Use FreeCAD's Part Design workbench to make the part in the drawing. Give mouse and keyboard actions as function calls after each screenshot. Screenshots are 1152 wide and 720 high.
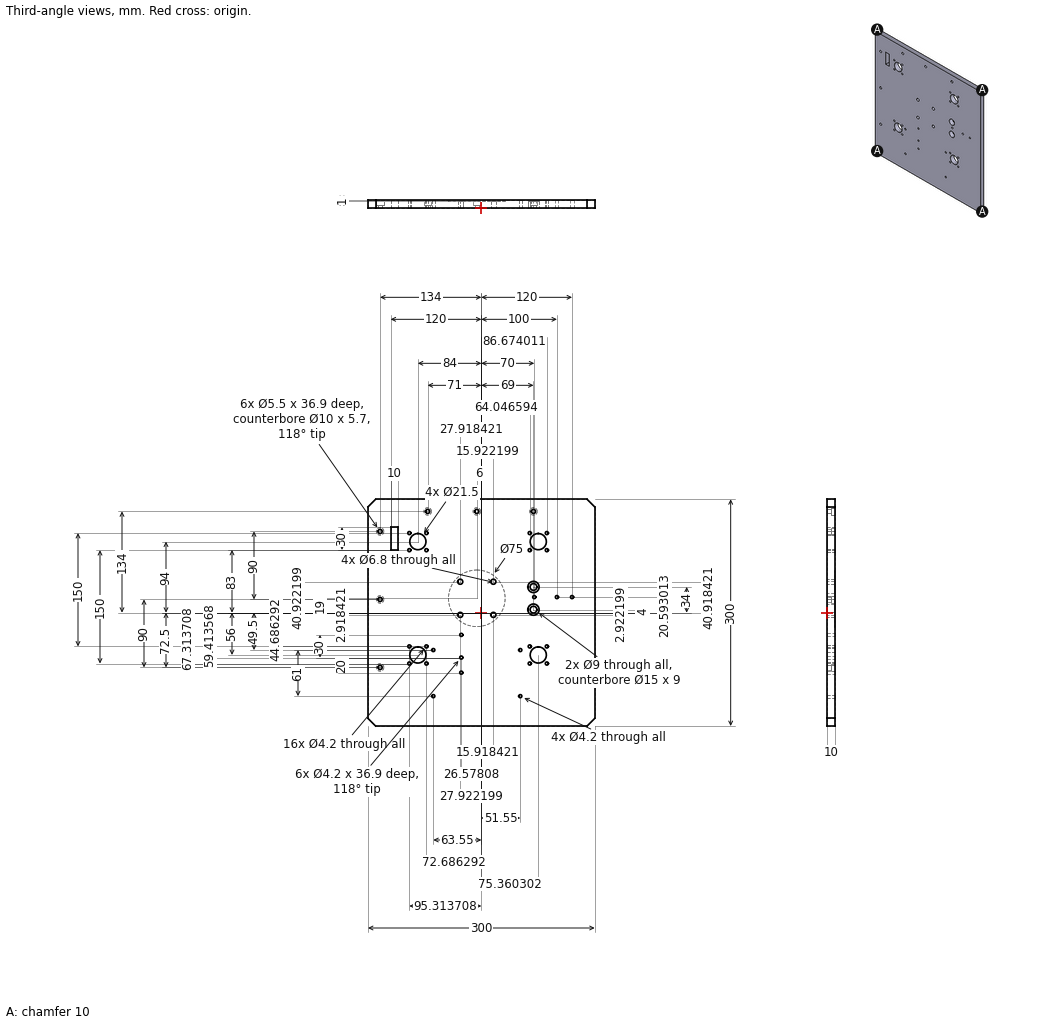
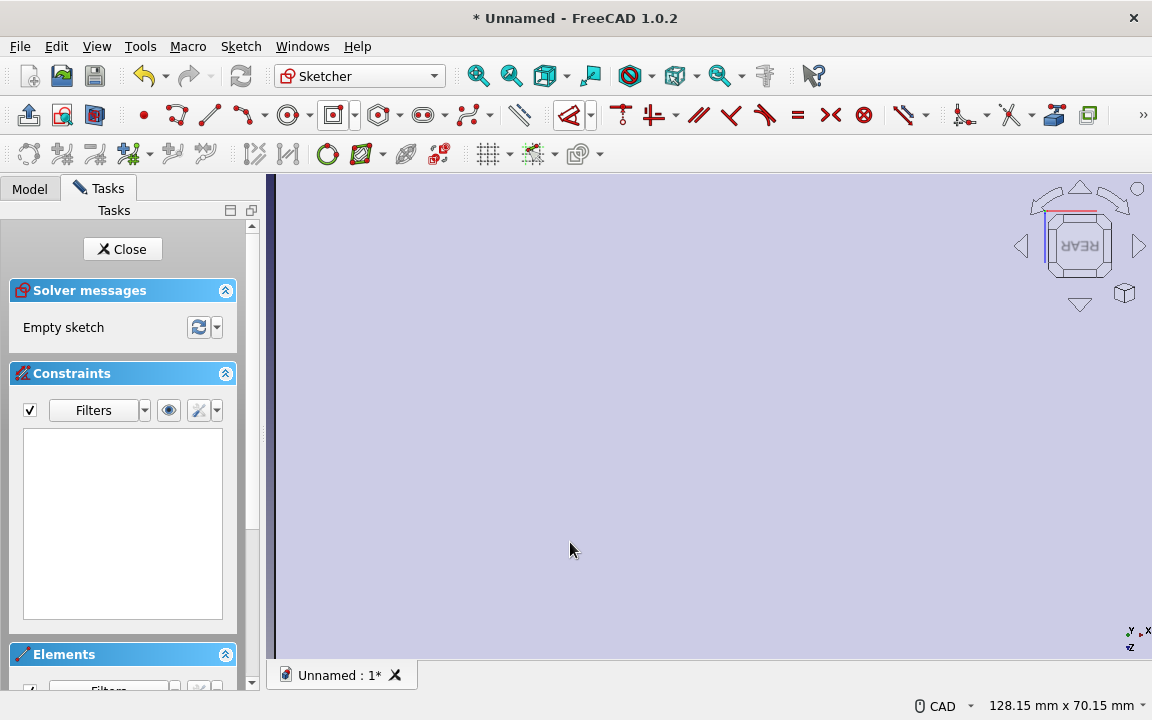
click(354, 116)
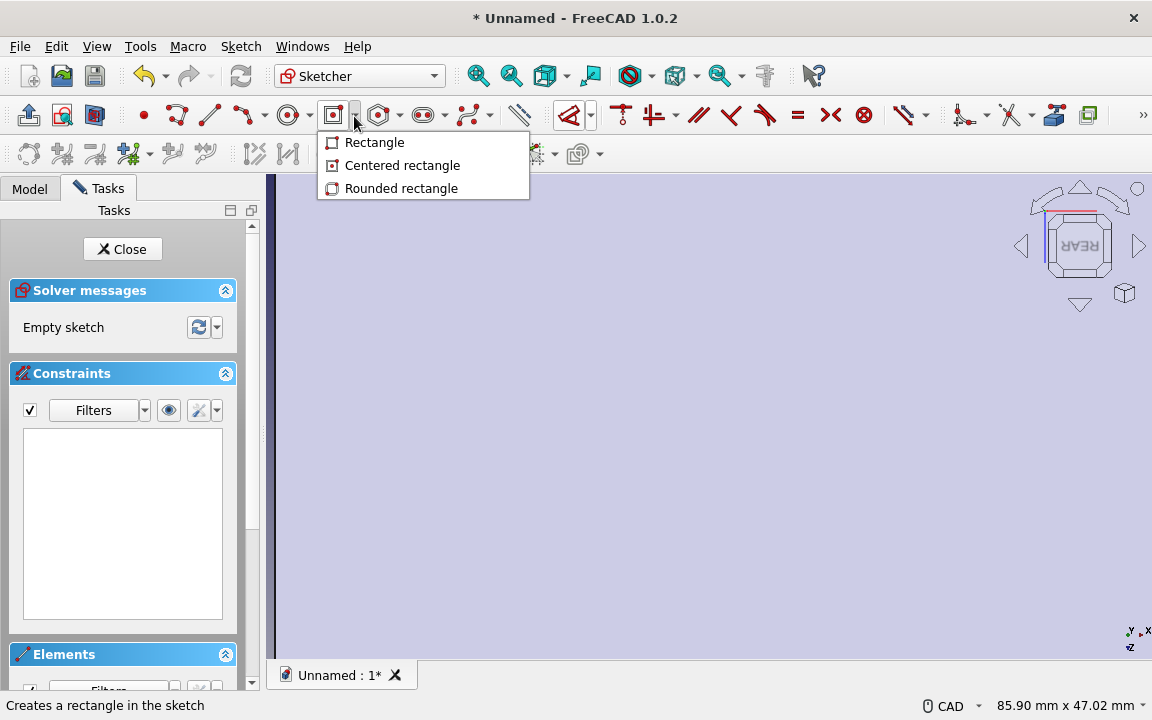
click(424, 142)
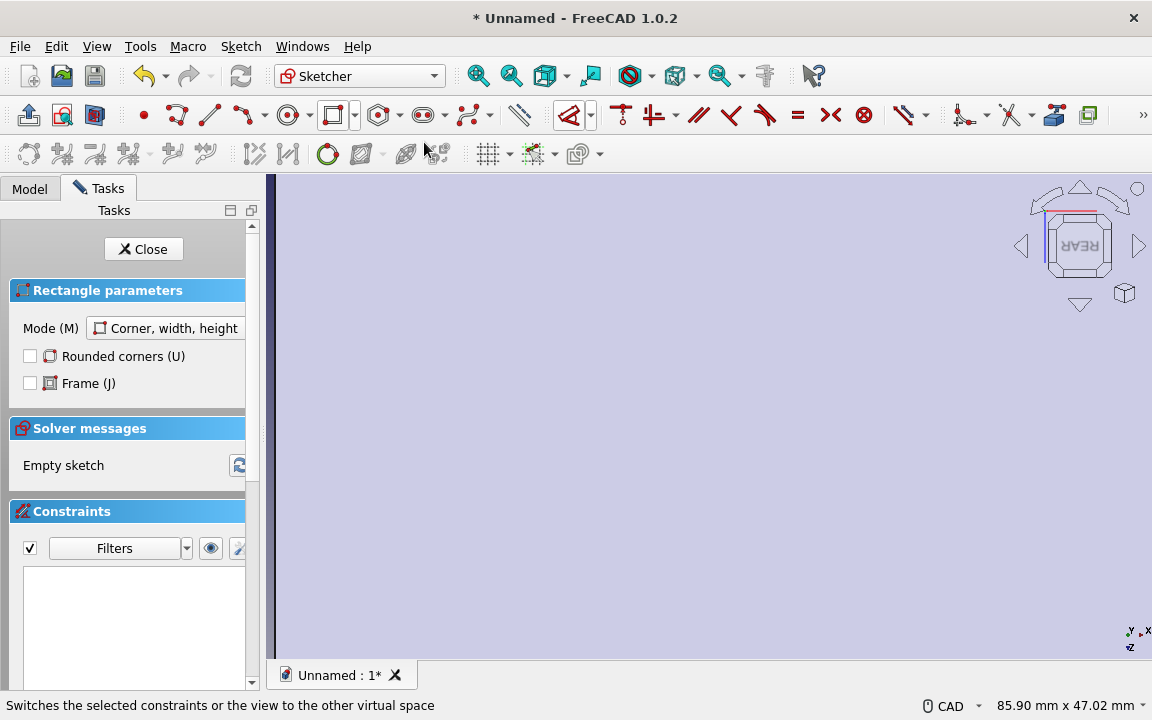
click(584, 259)
move(687, 569)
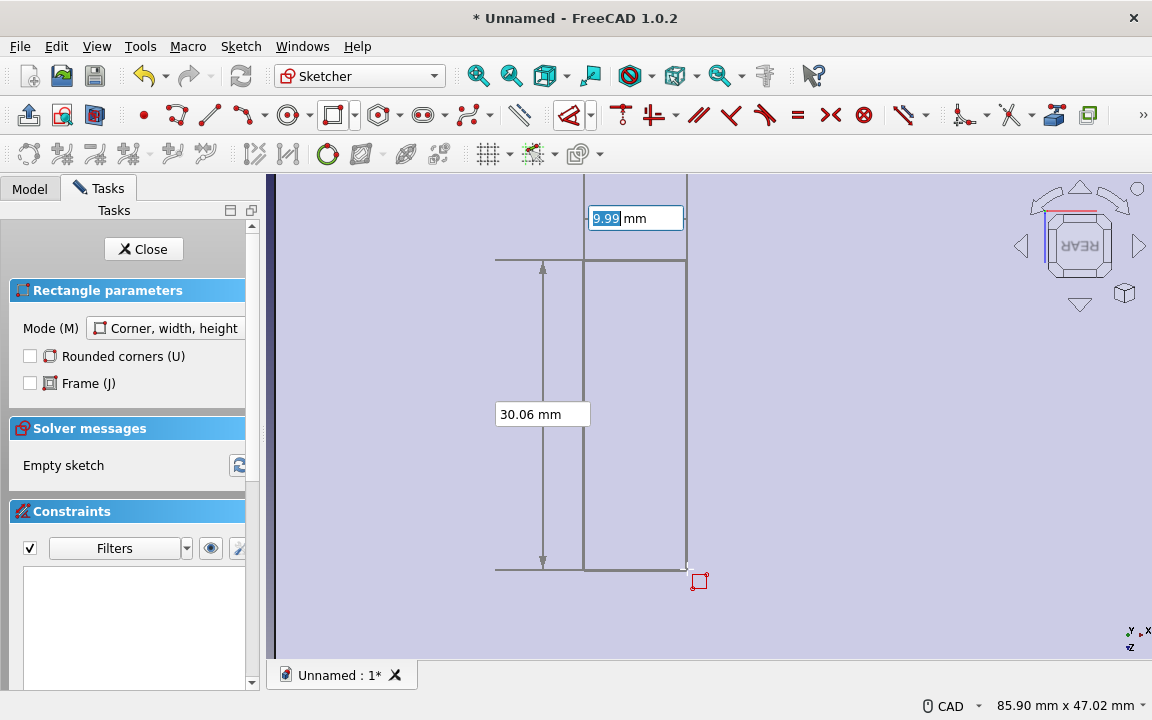
text(10)
key(Tab)
text(30)
key(Return)
key(Escape)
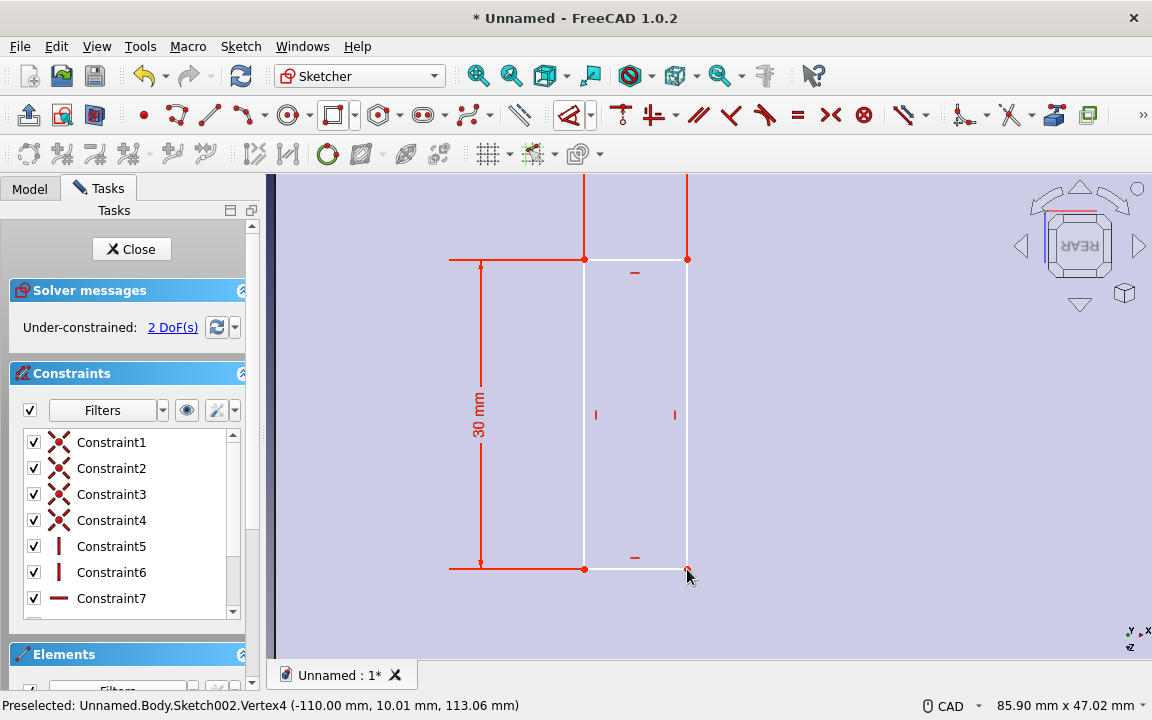
click(584, 260)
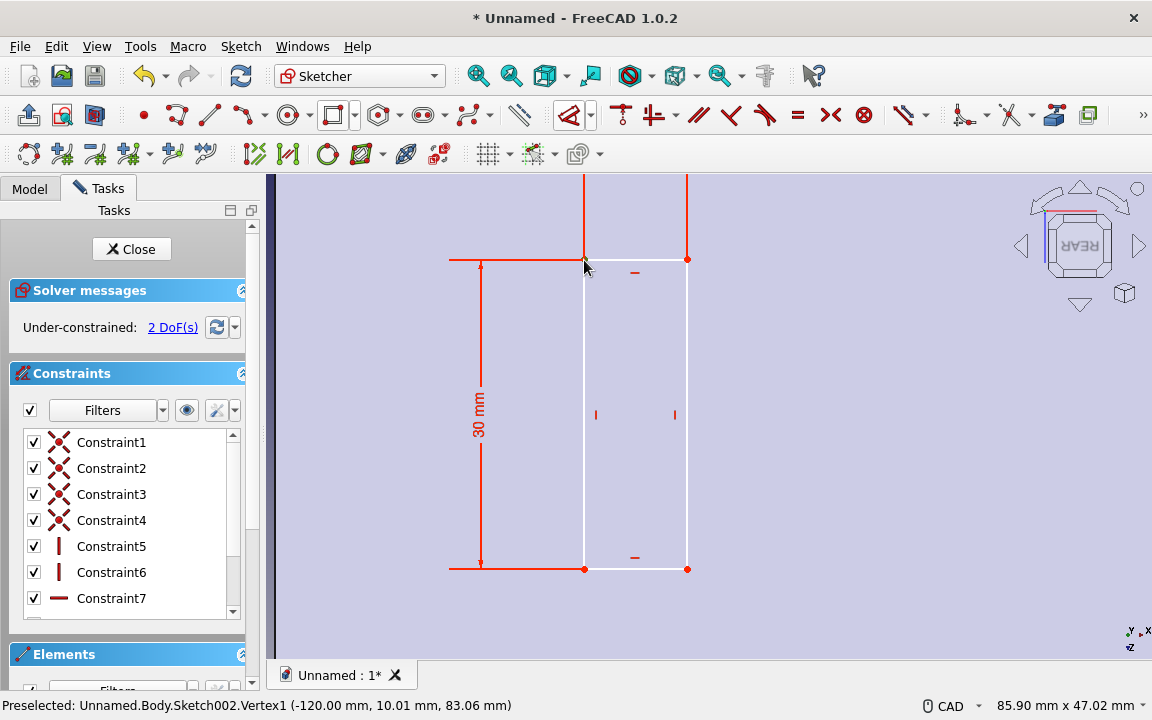
key(i)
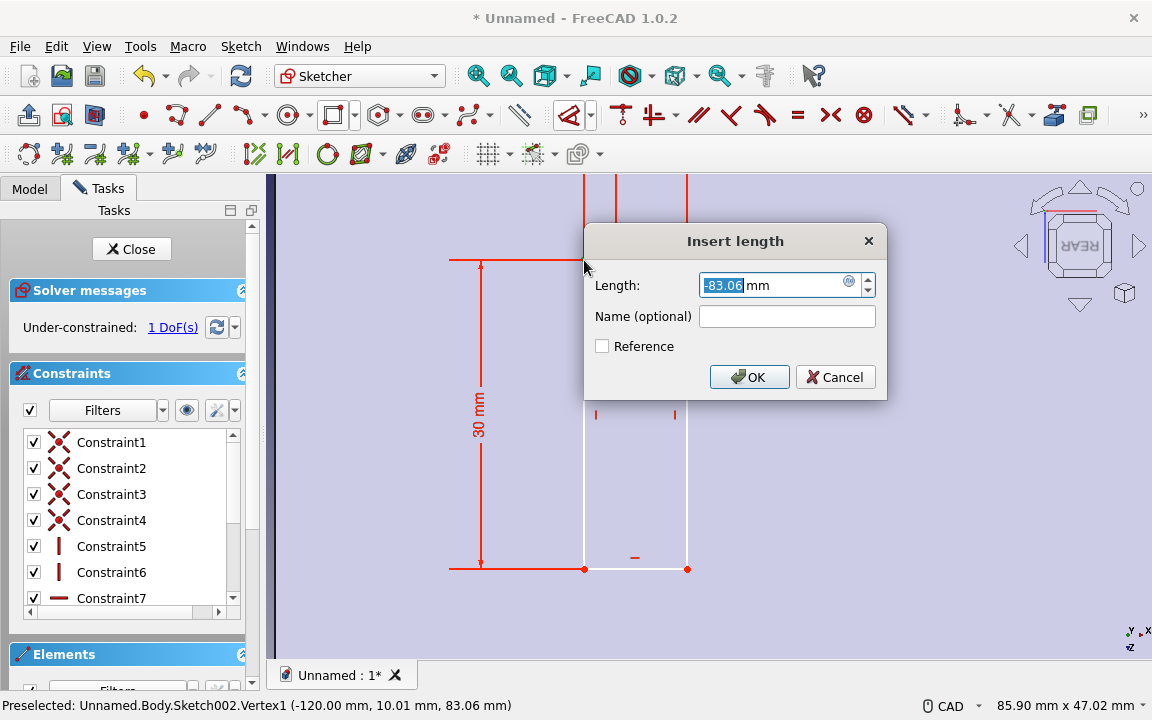
text(-83)
key(Return)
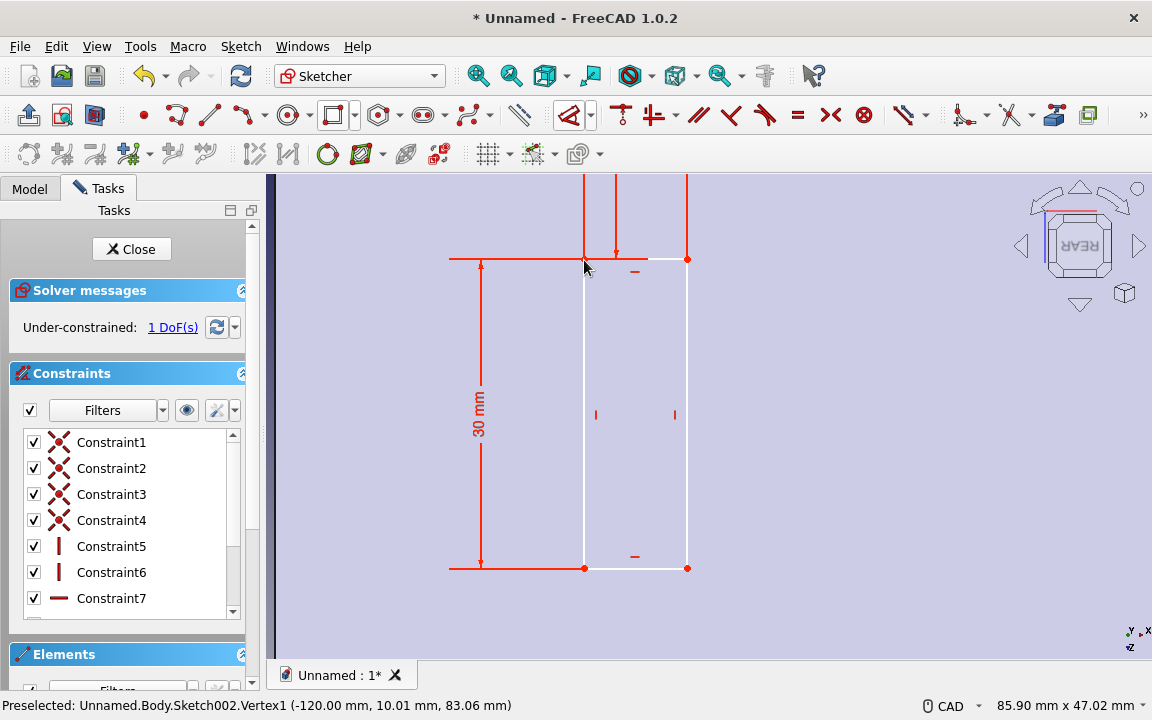
click(584, 259)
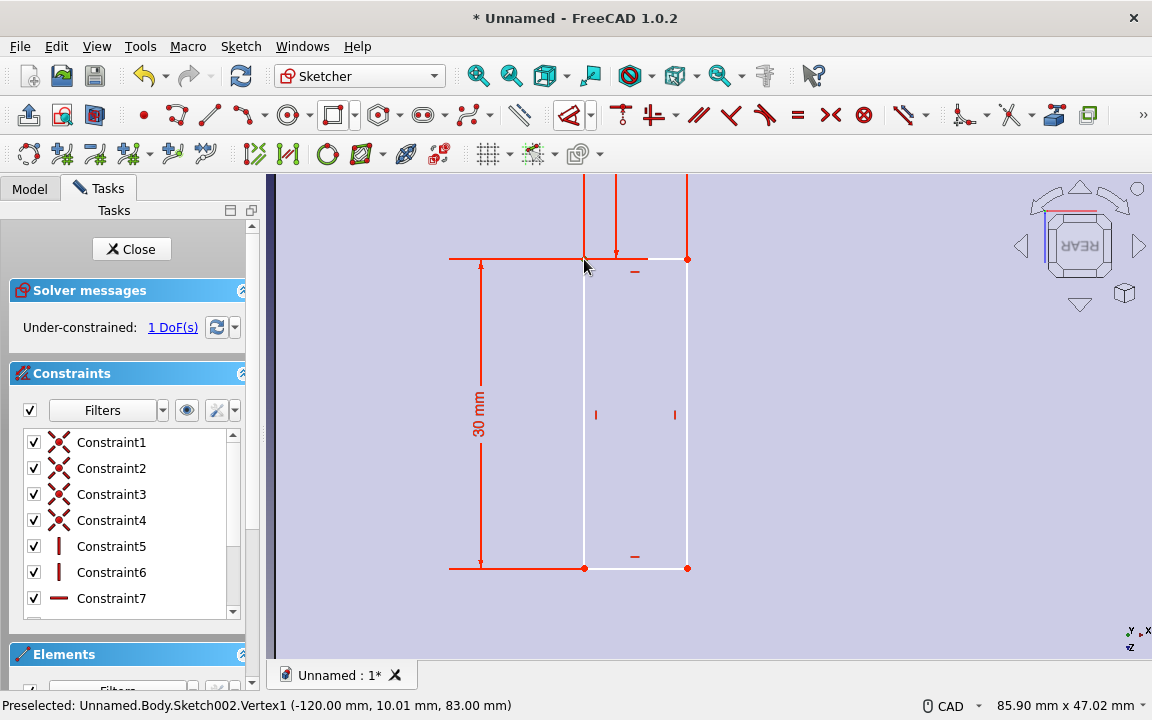
click(590, 116)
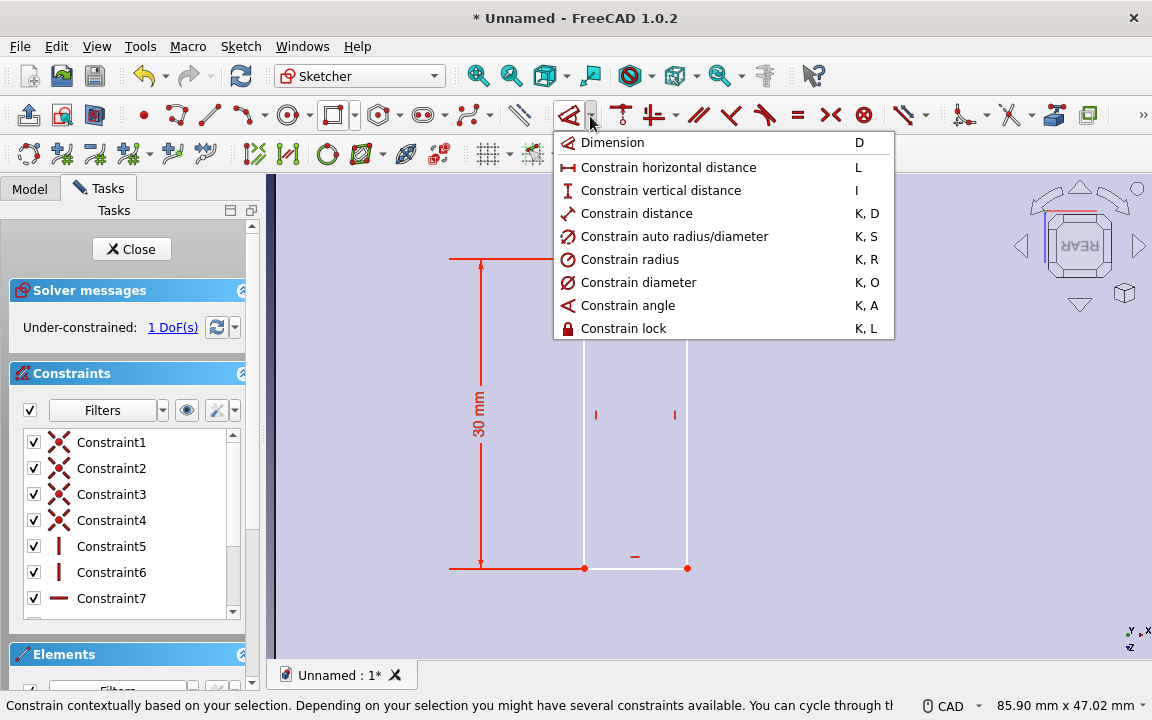
click(724, 168)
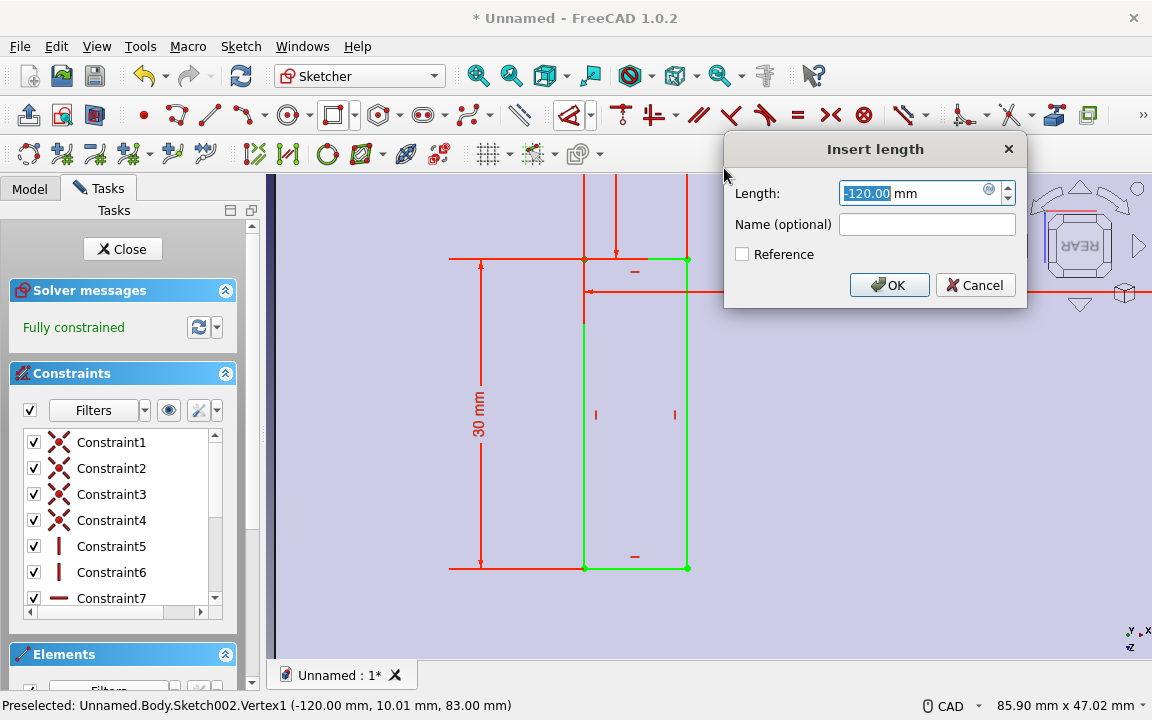
text(-120)
key(Return)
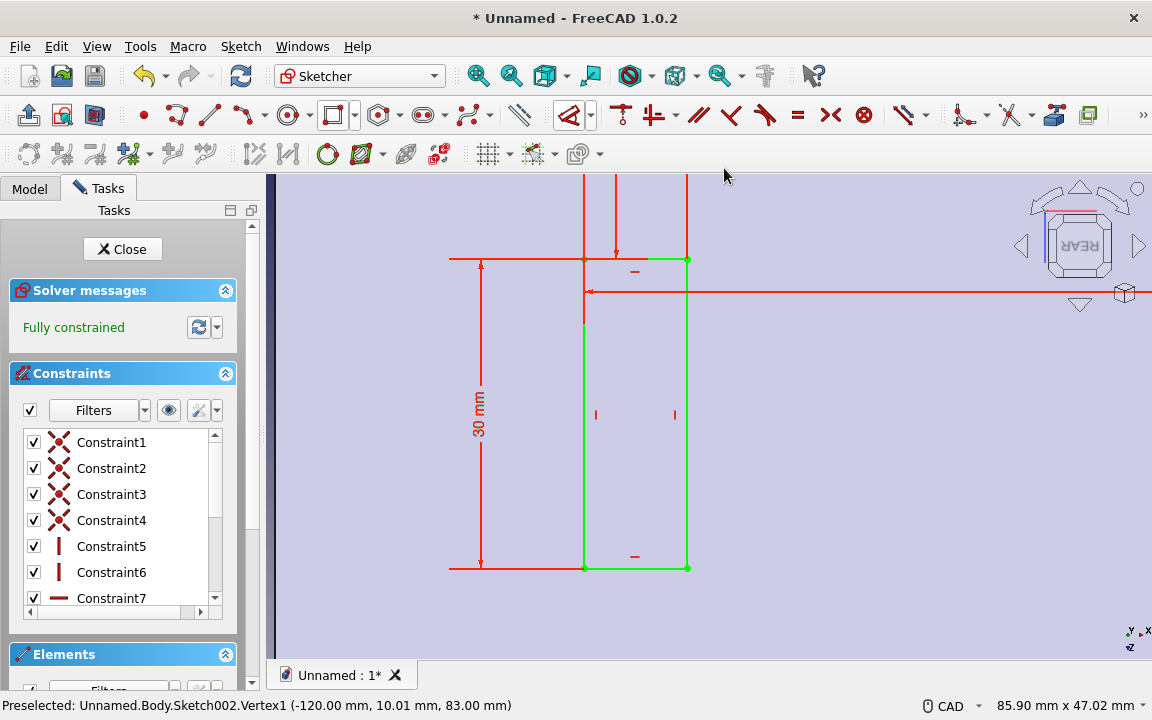
click(123, 249)